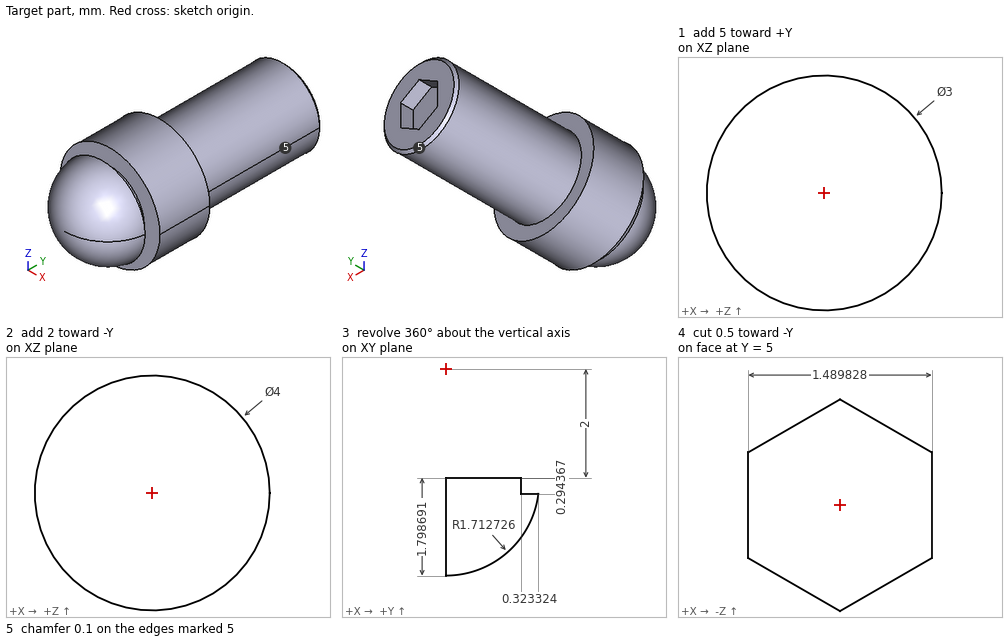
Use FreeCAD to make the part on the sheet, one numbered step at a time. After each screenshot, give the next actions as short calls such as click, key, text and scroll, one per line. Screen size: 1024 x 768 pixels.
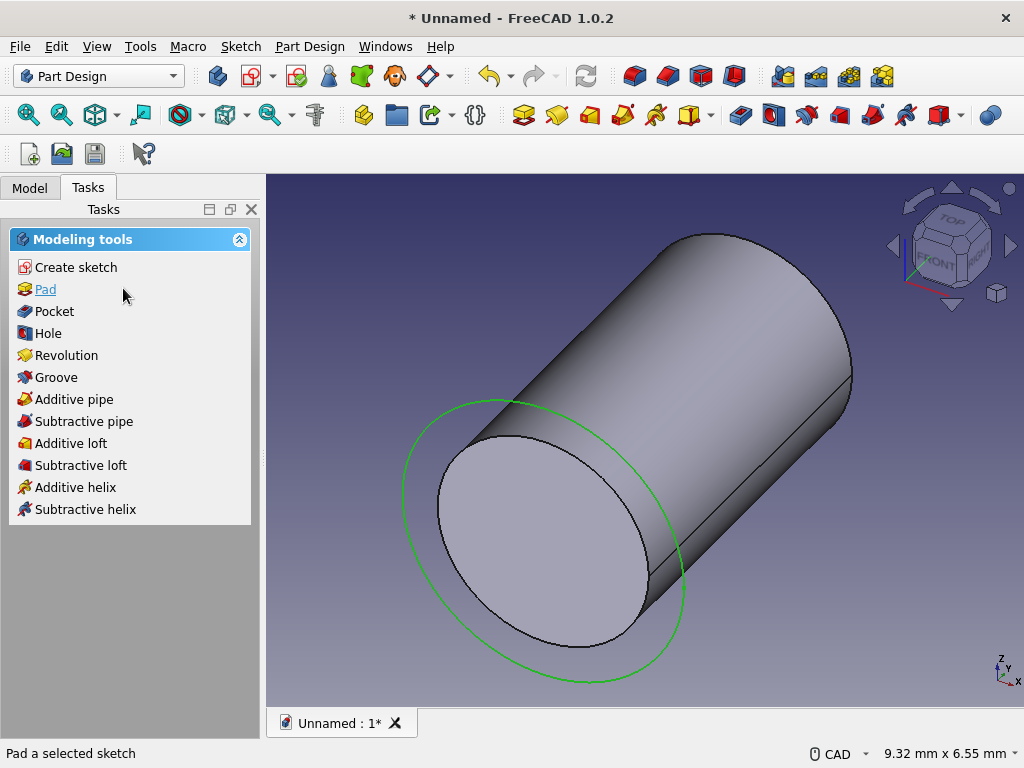
click(524, 116)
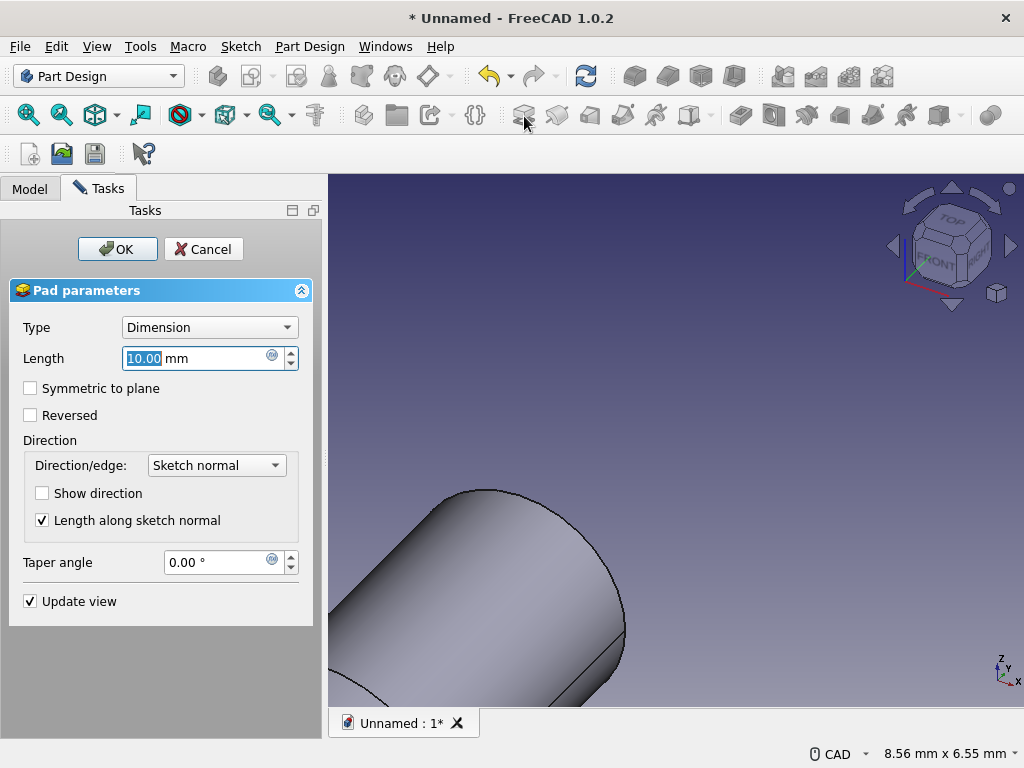
text(2)
key(Tab)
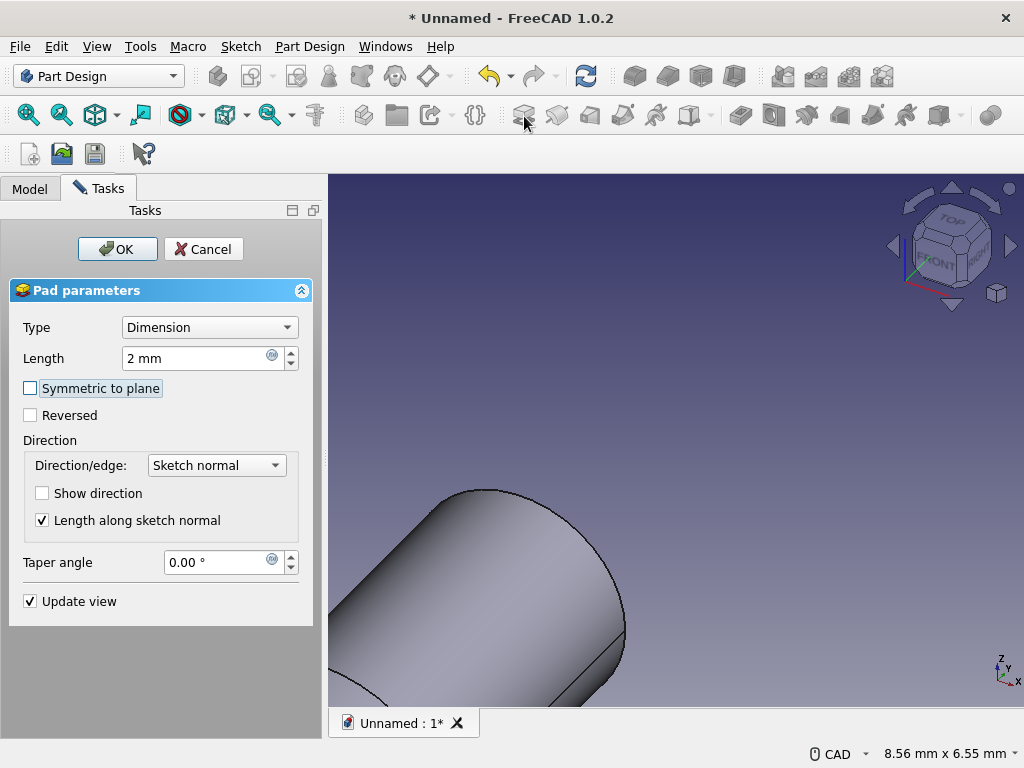
click(118, 249)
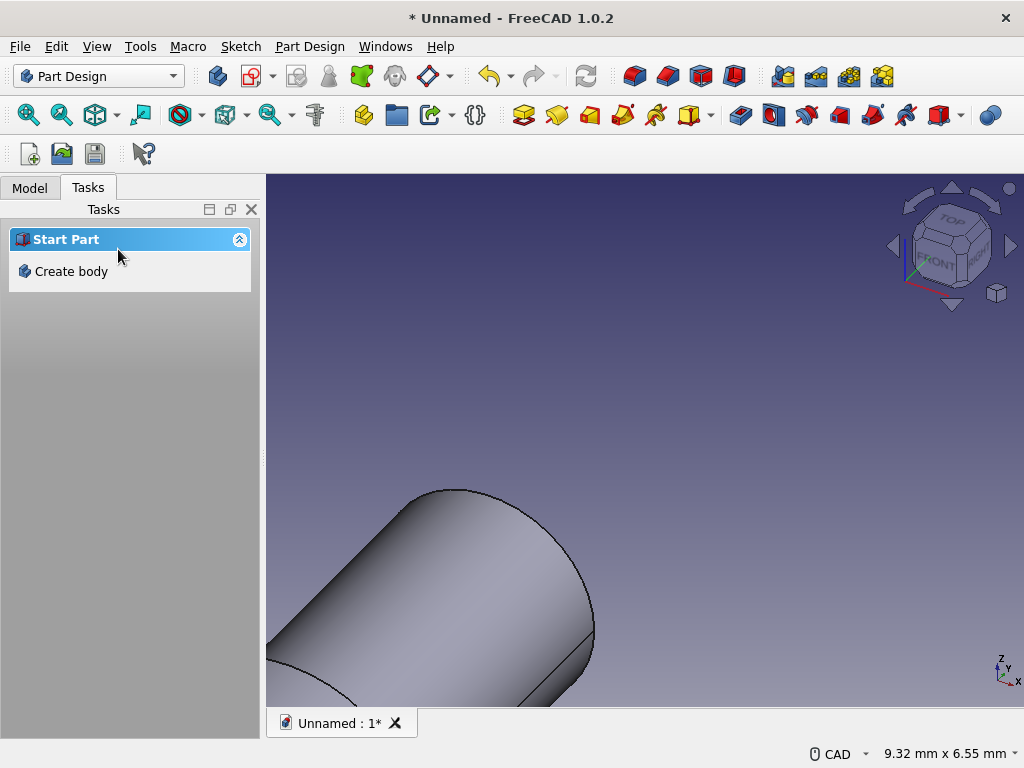
click(29, 116)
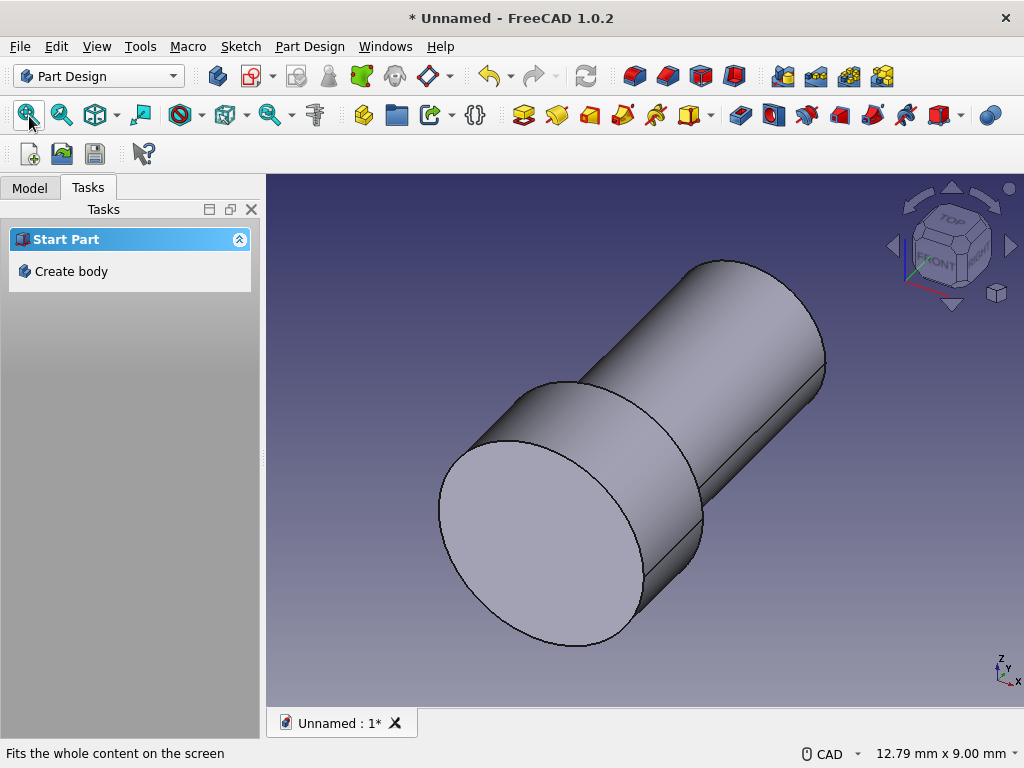
click(250, 76)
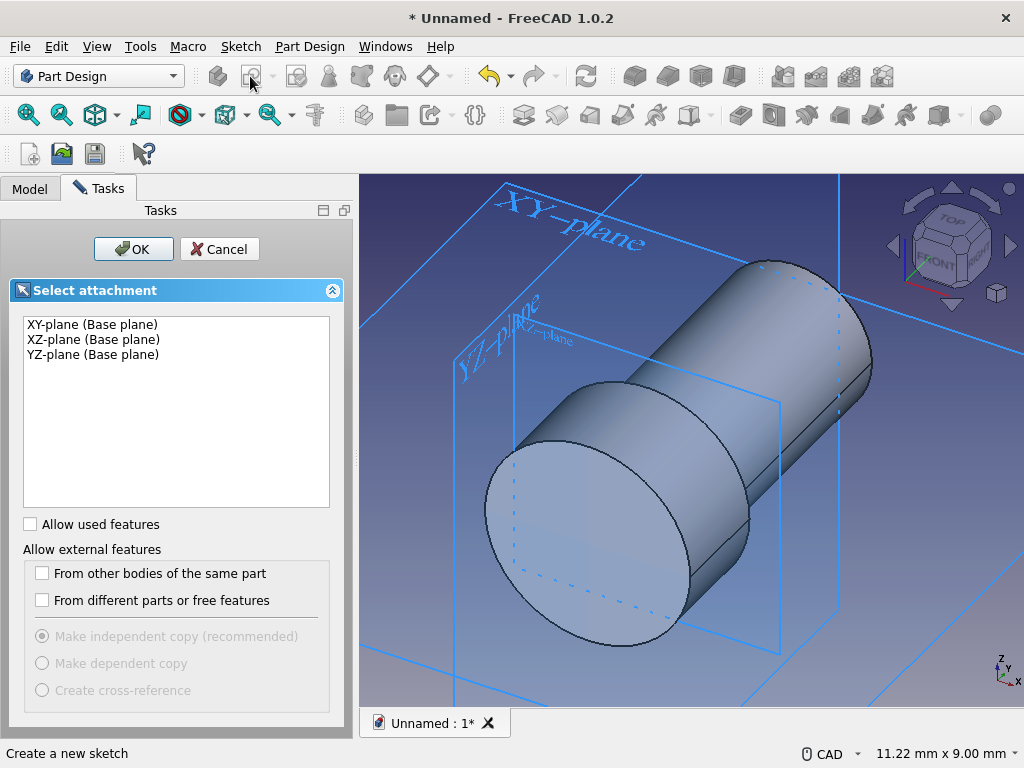
click(84, 324)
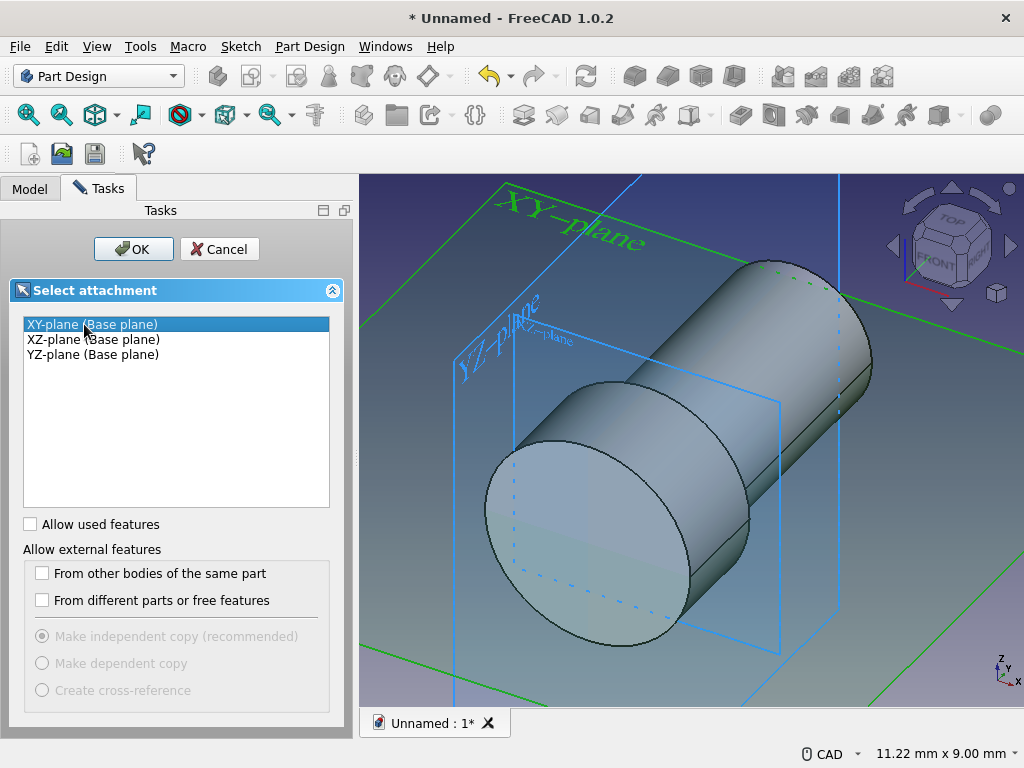
click(134, 249)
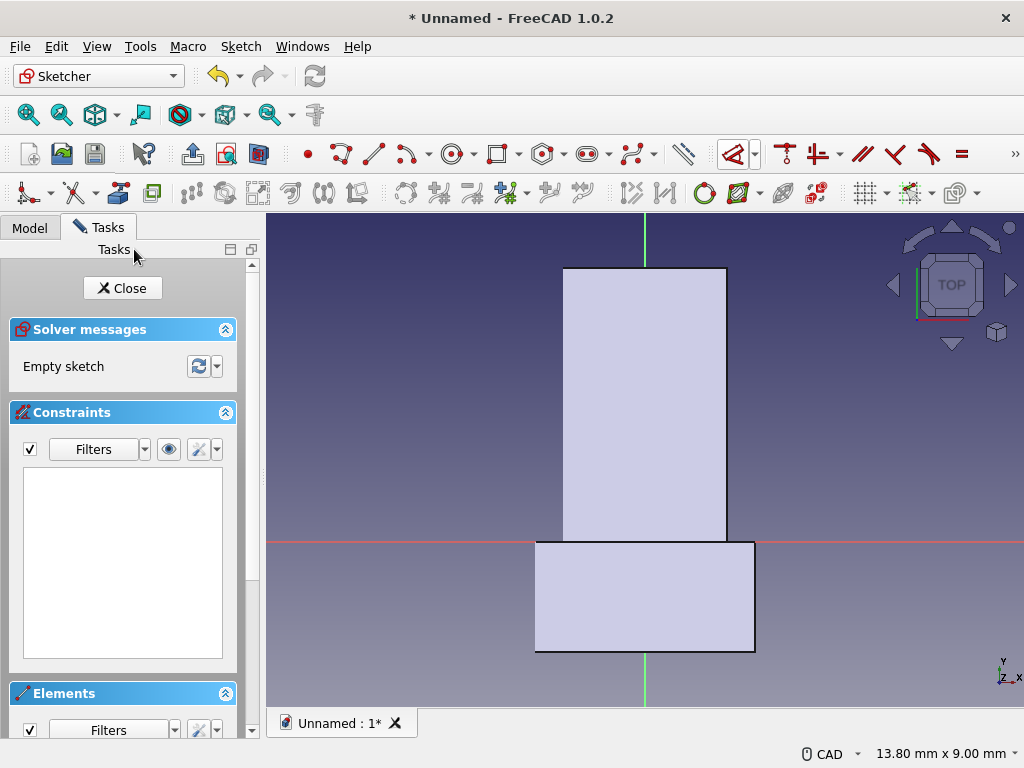
click(259, 154)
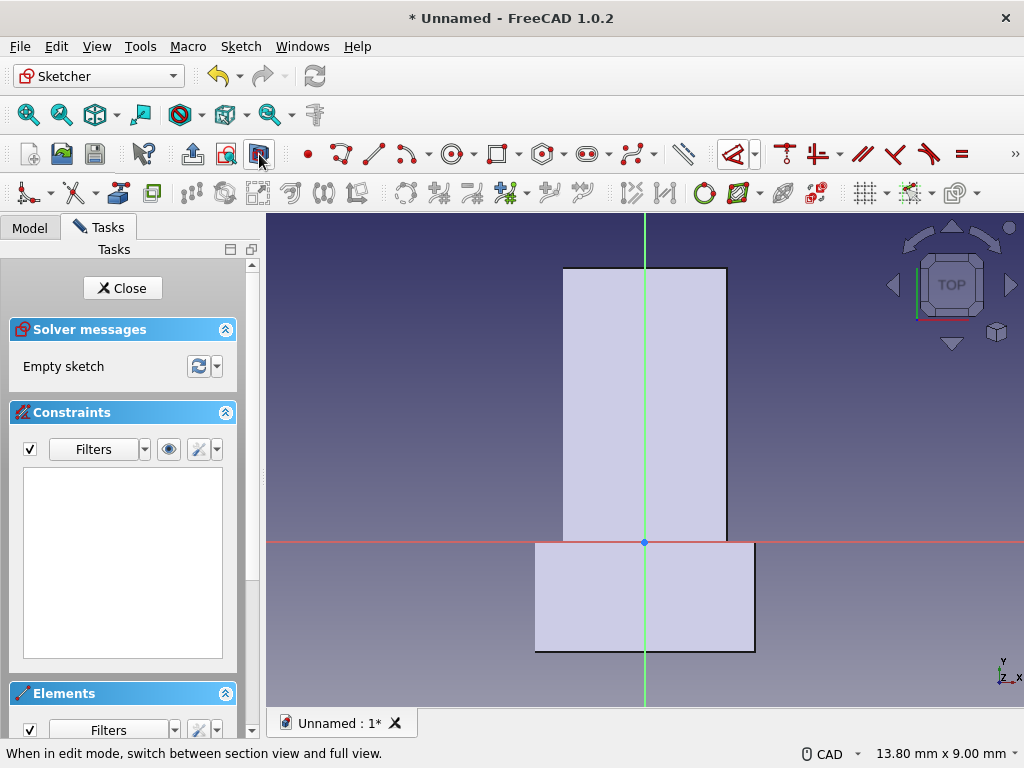
scroll(576, 460, down, 5)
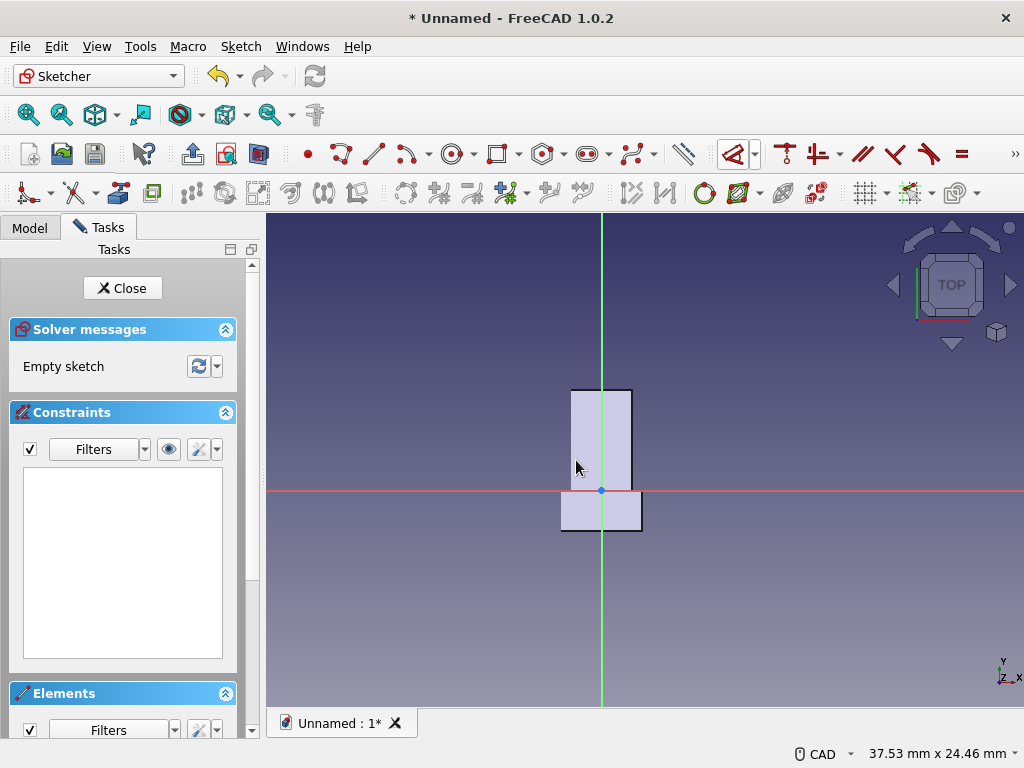
scroll(633, 552, up, 7)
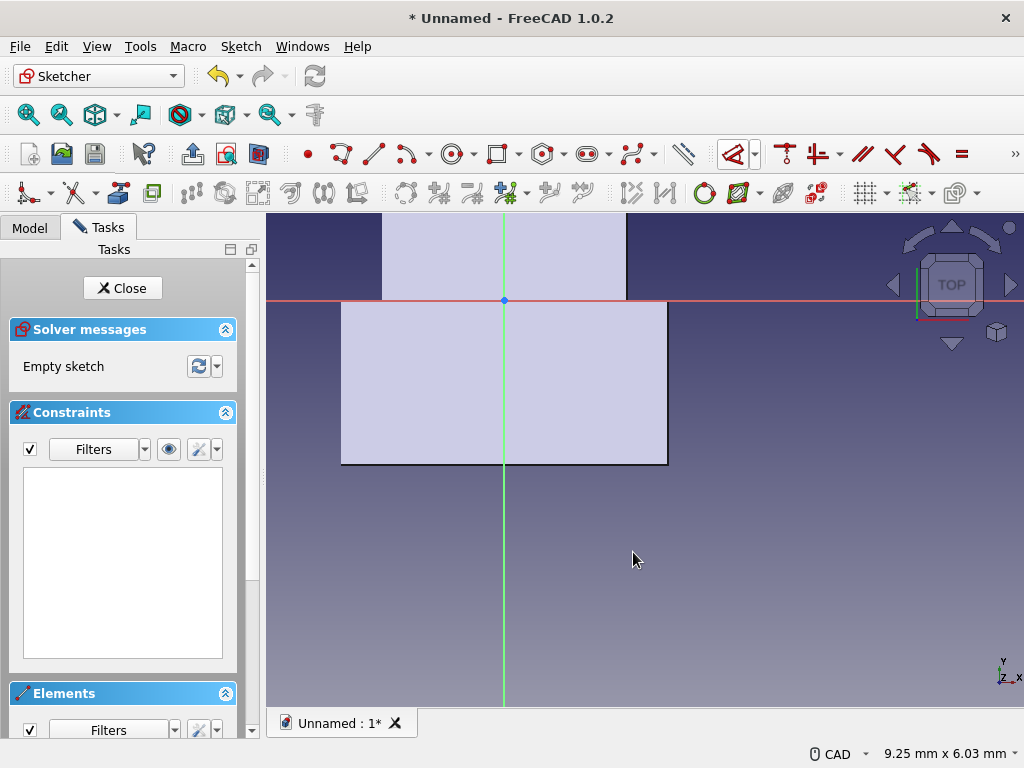
click(341, 154)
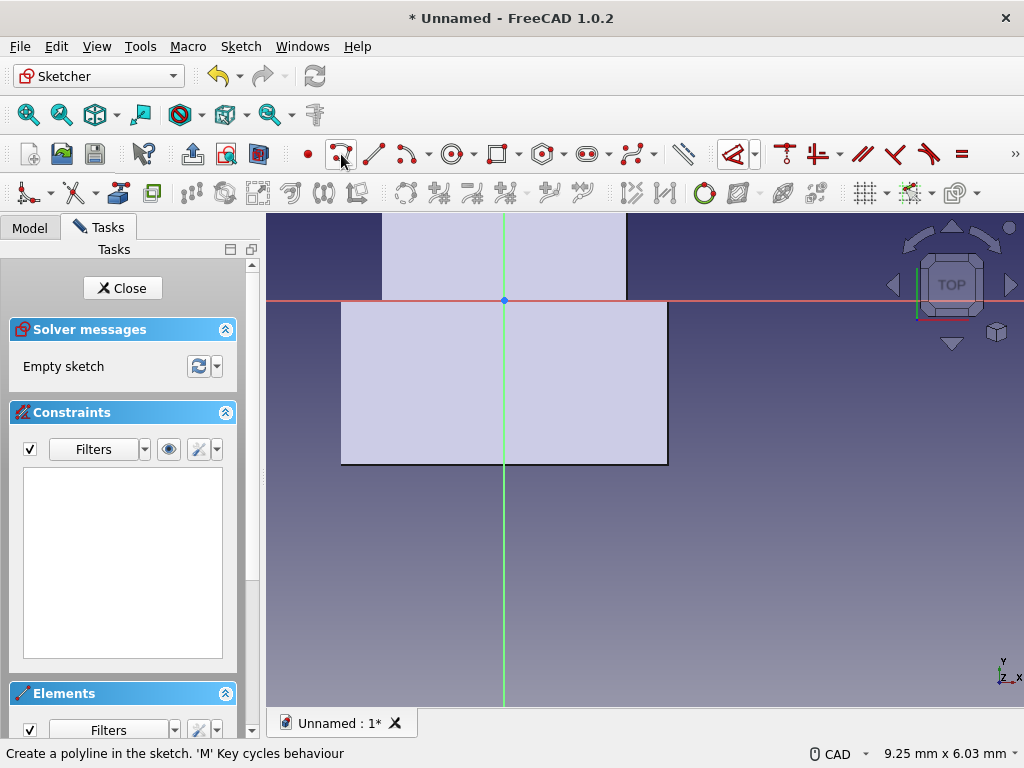
click(643, 489)
click(617, 489)
click(617, 465)
click(504, 465)
click(513, 612)
right_click(513, 612)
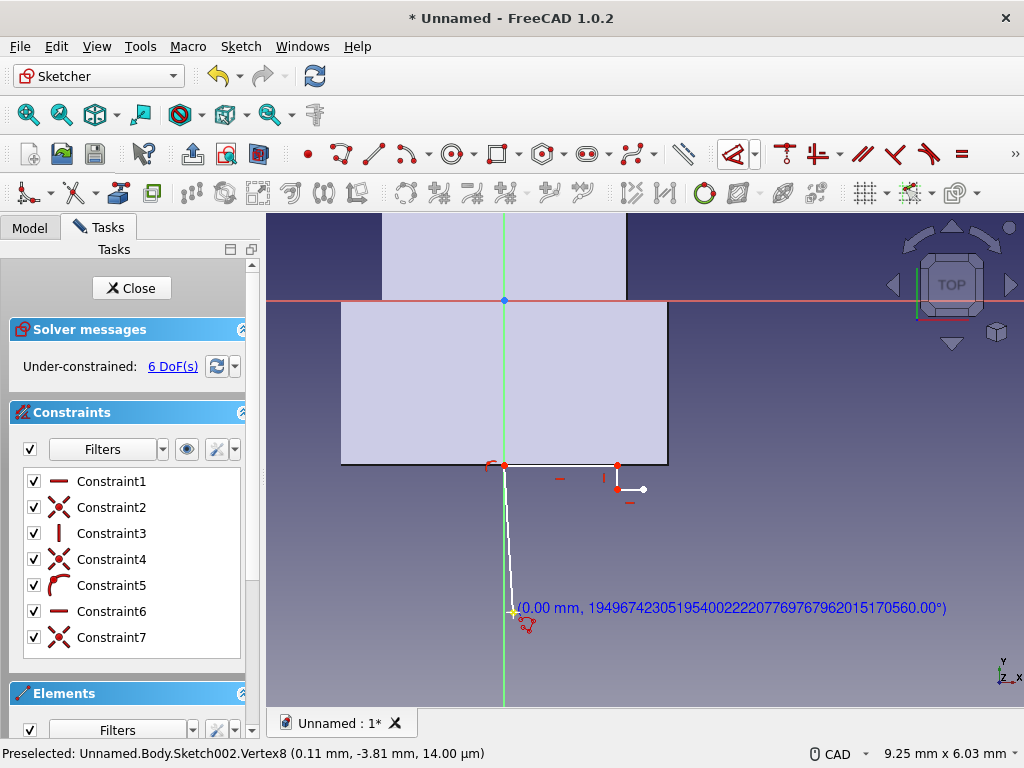
click(428, 154)